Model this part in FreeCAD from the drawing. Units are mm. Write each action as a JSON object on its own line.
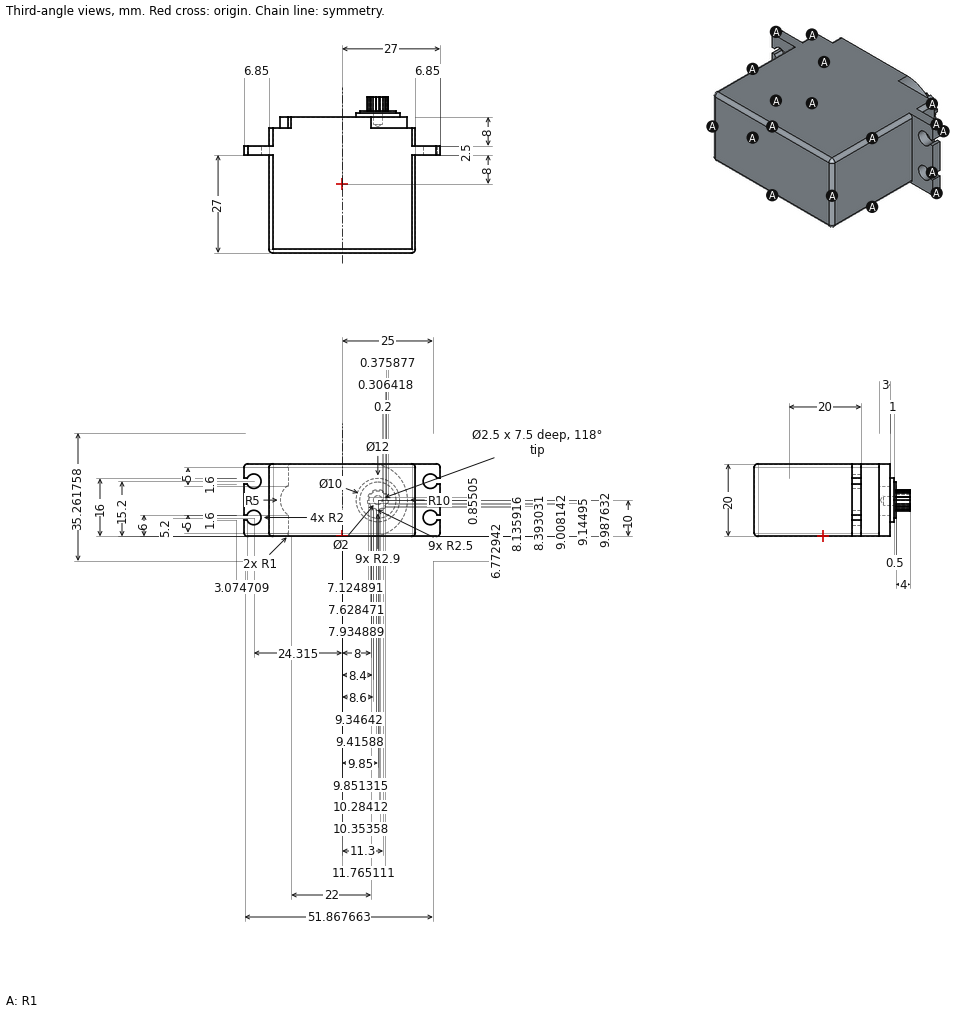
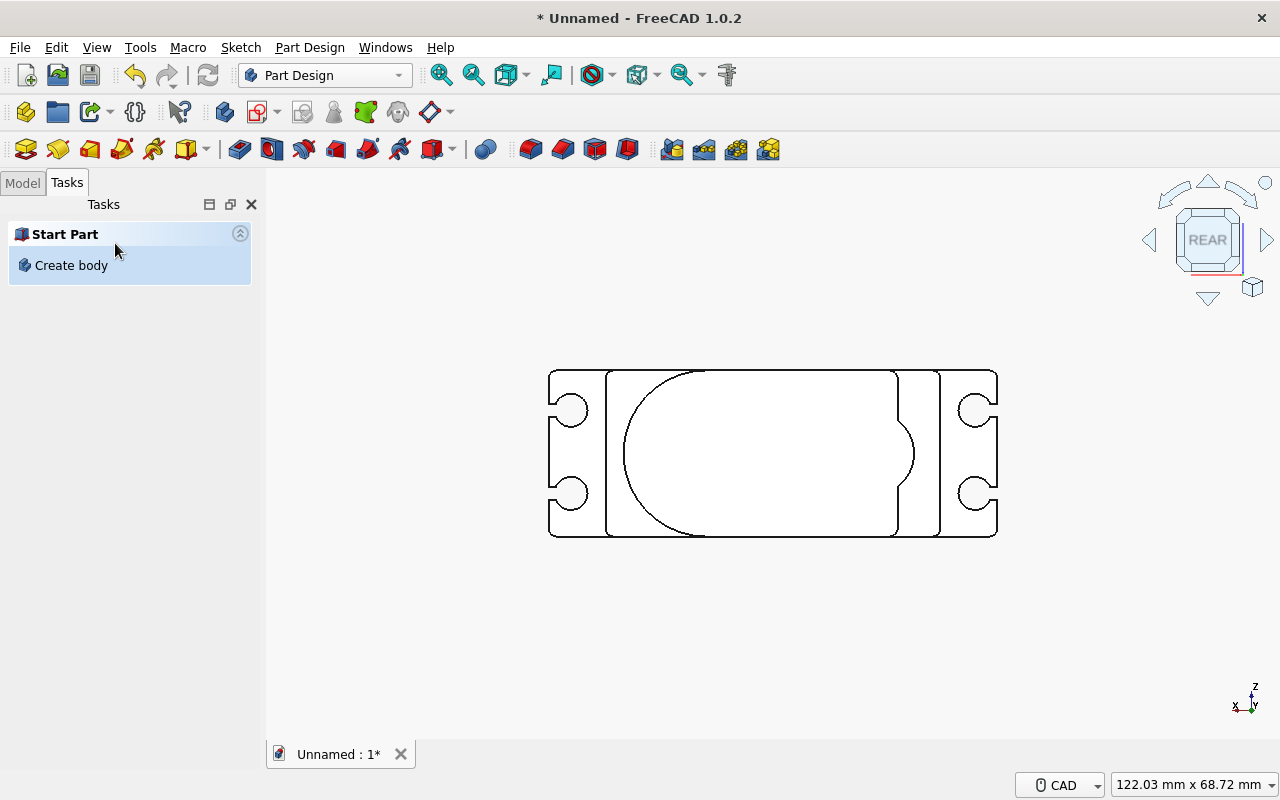
{"action": "left_click", "coordinate": [442, 76]}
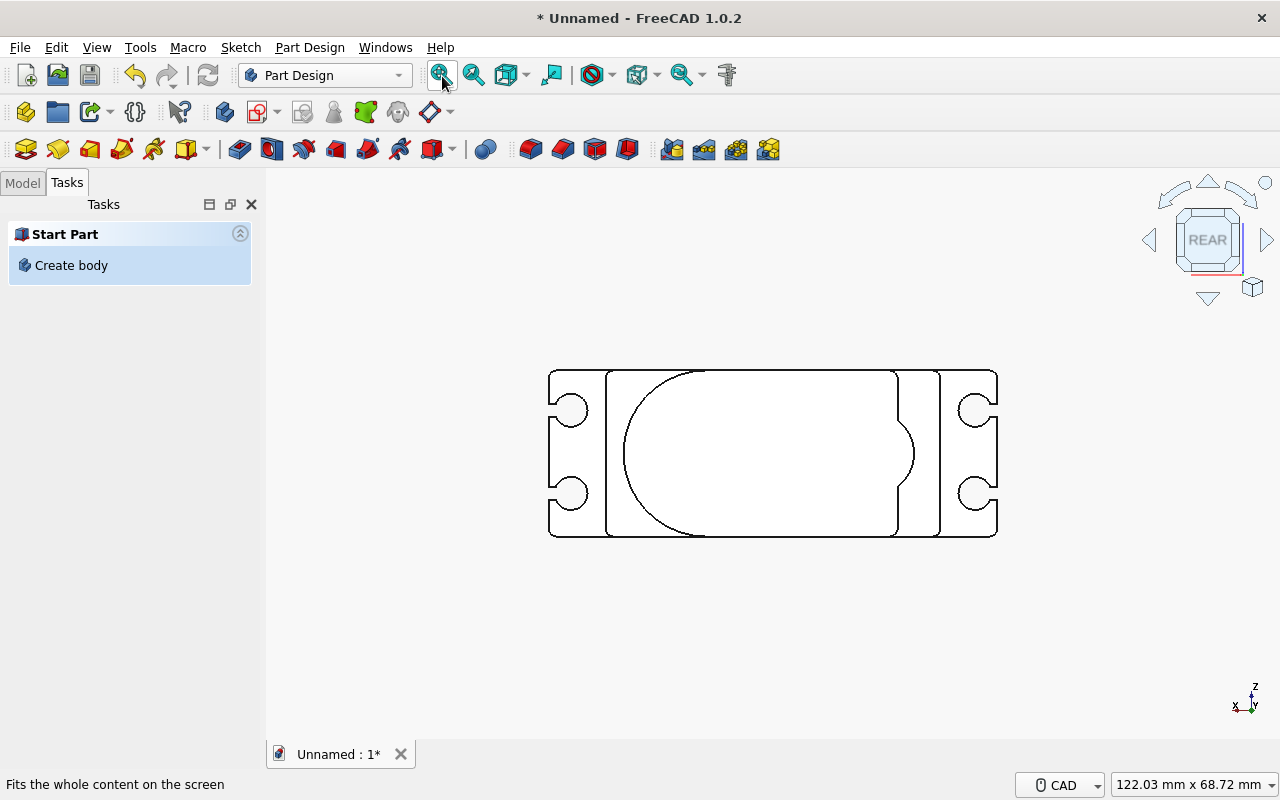
{"action": "left_click", "coordinate": [727, 452]}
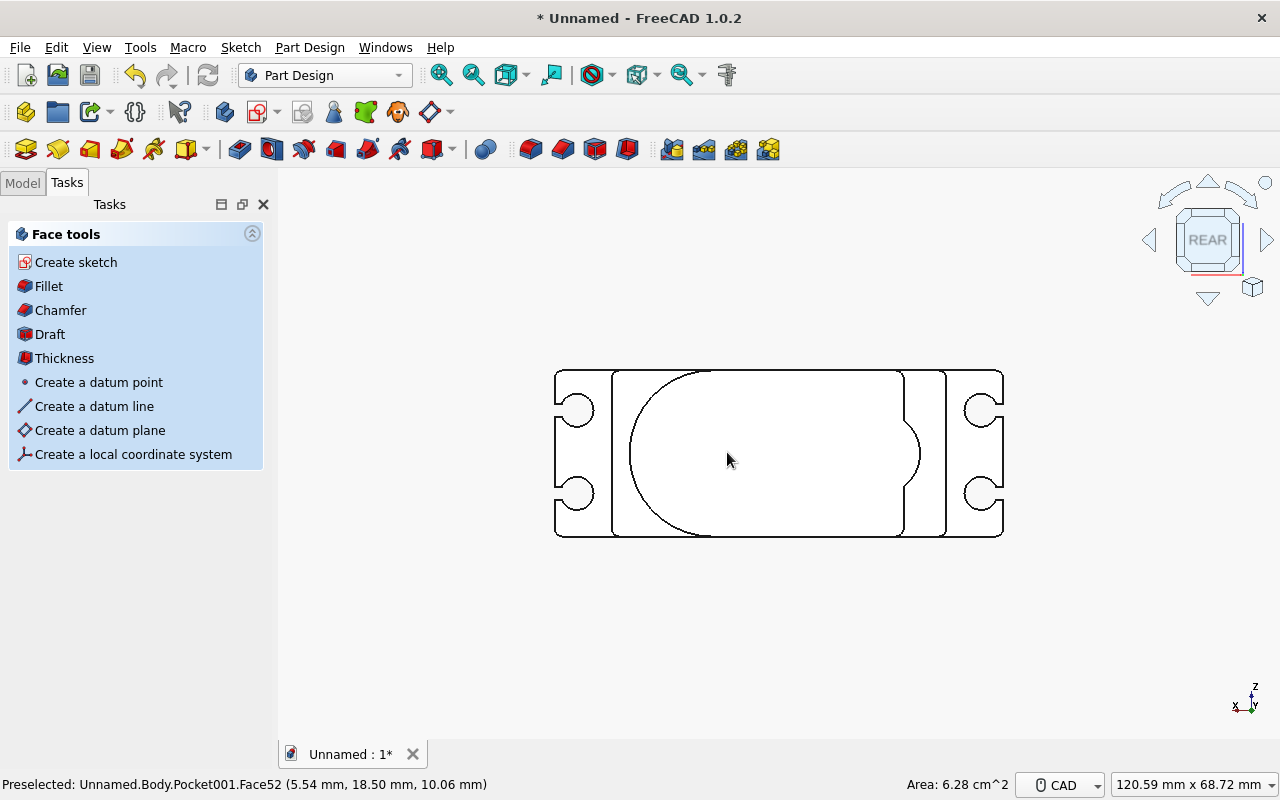
{"action": "left_click", "coordinate": [258, 112]}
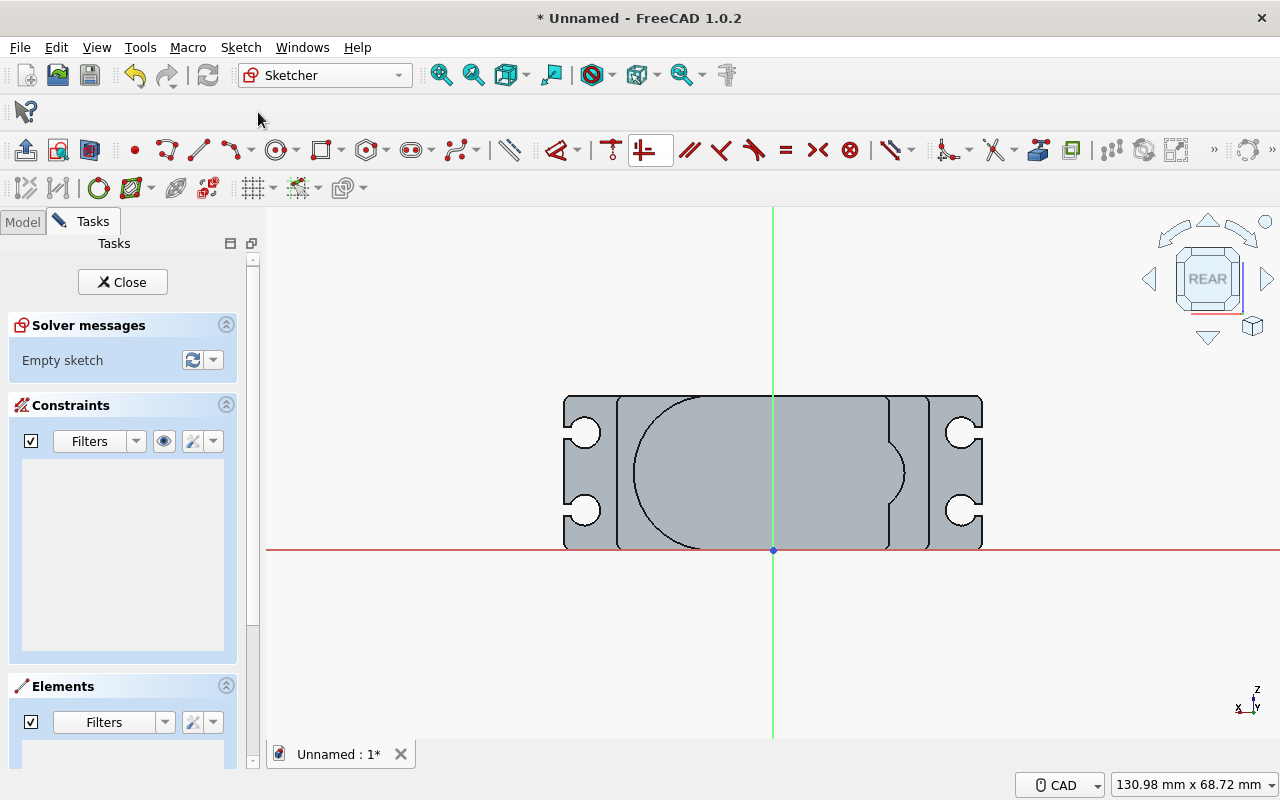
{"action": "scroll", "coordinate": [716, 497], "scroll_direction": "up", "scroll_amount": 5}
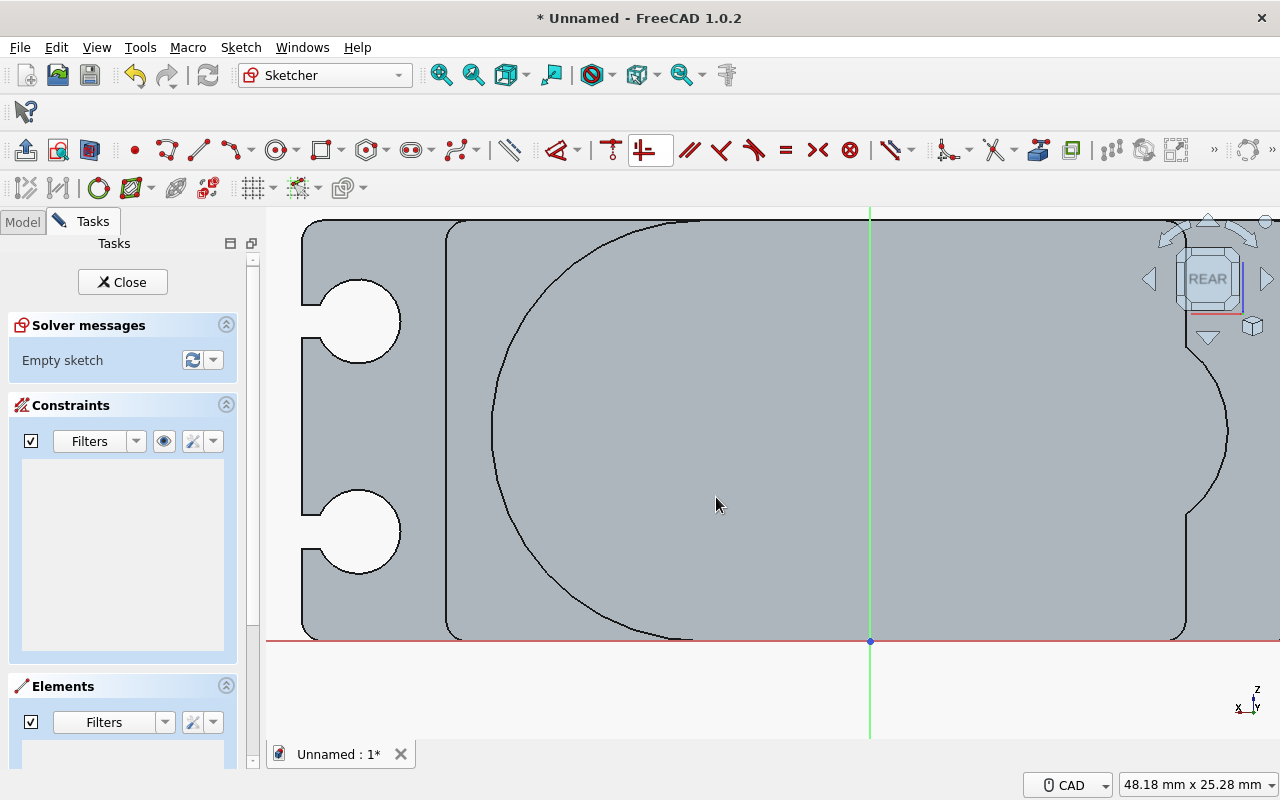
{"action": "left_click", "coordinate": [276, 150]}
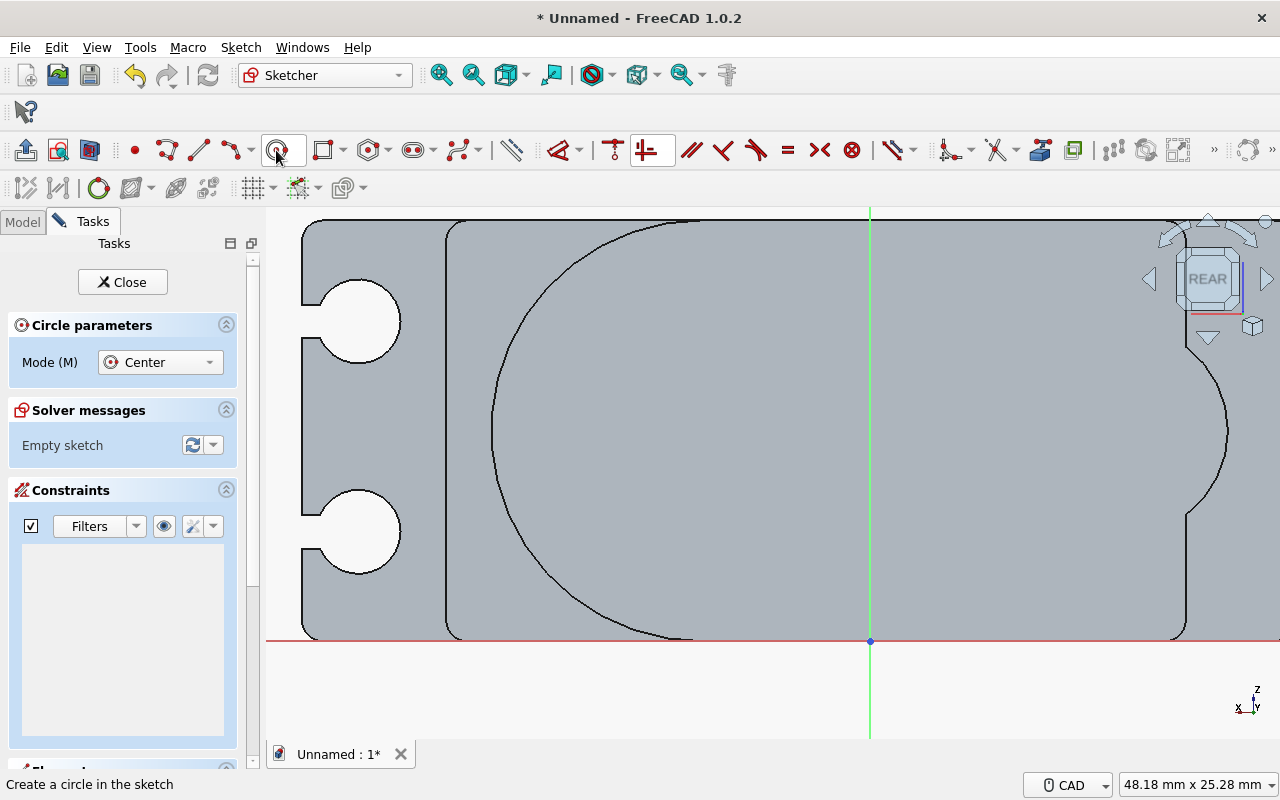
{"action": "left_click", "coordinate": [663, 431]}
{"action": "mouse_move", "coordinate": [752, 342]}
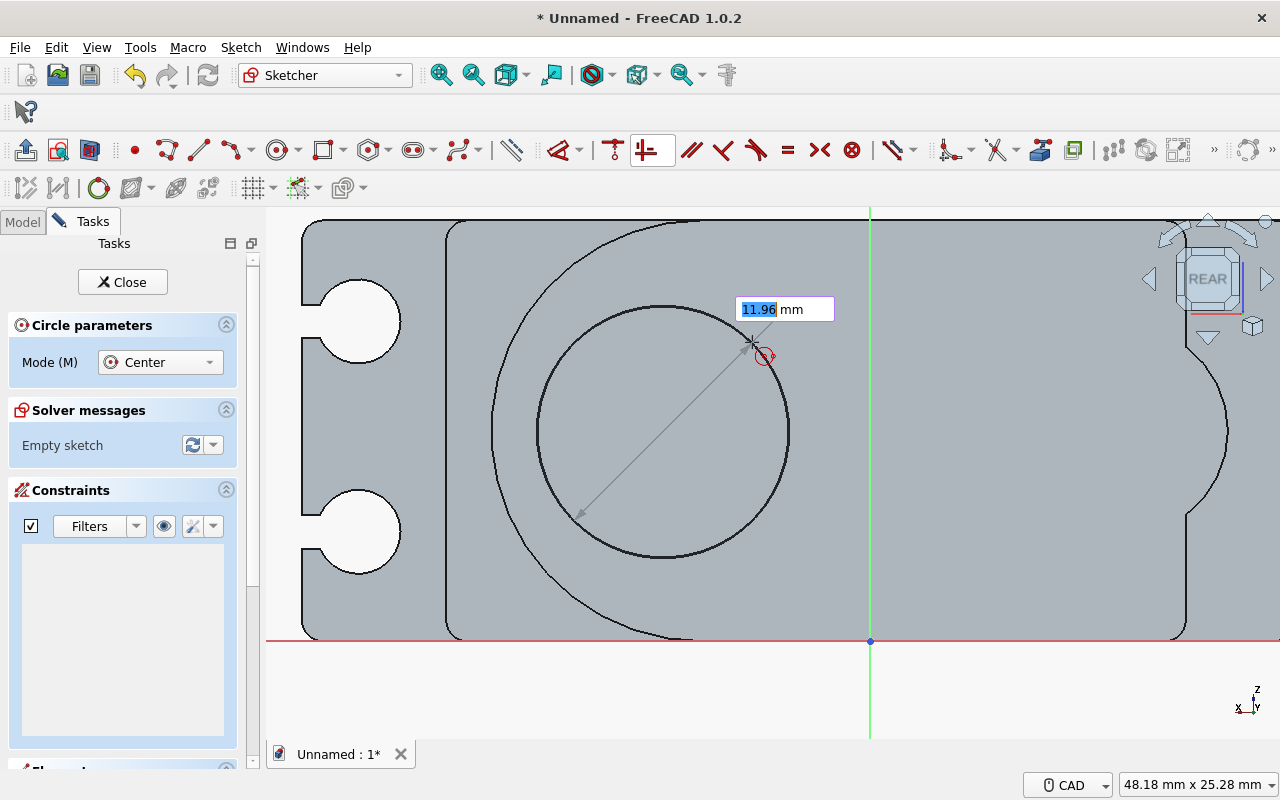
{"action": "type", "text": "12"}
{"action": "key", "text": "Return"}
{"action": "key", "text": "Escape"}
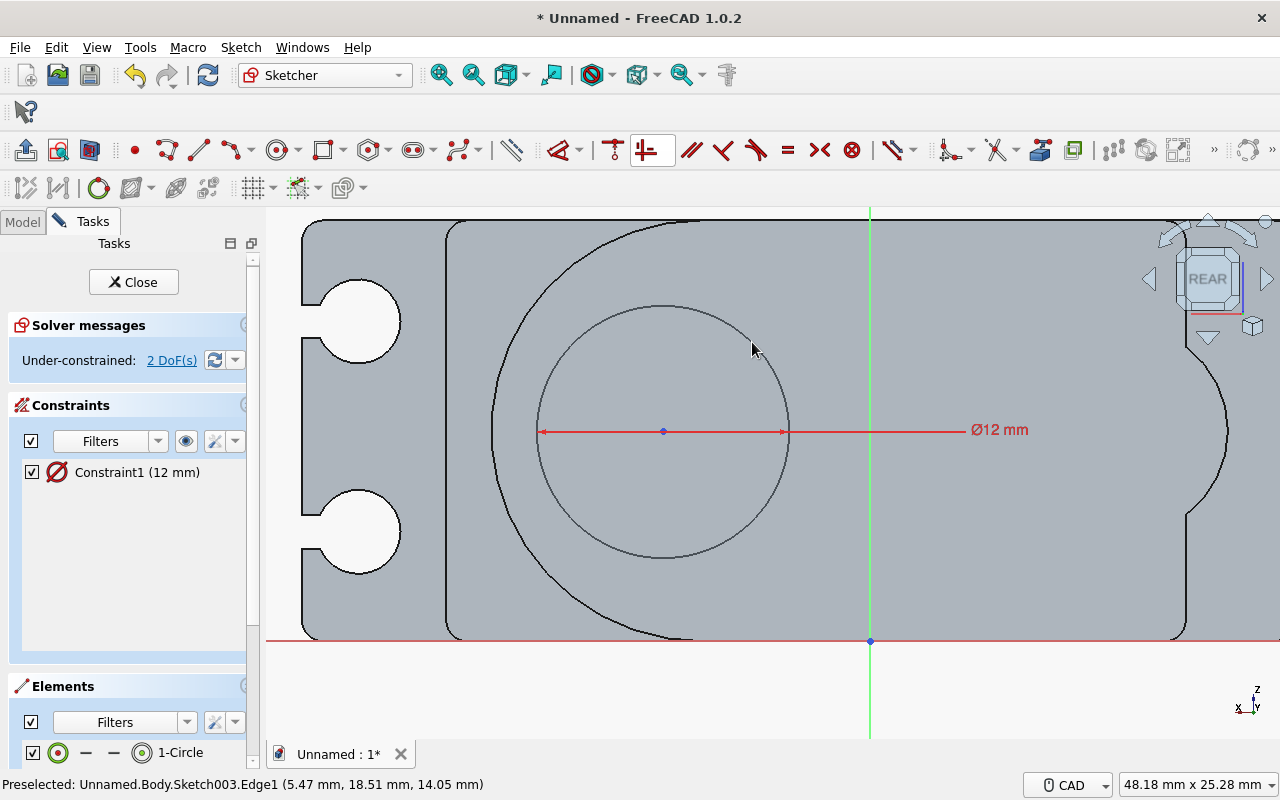
{"action": "left_click", "coordinate": [558, 150]}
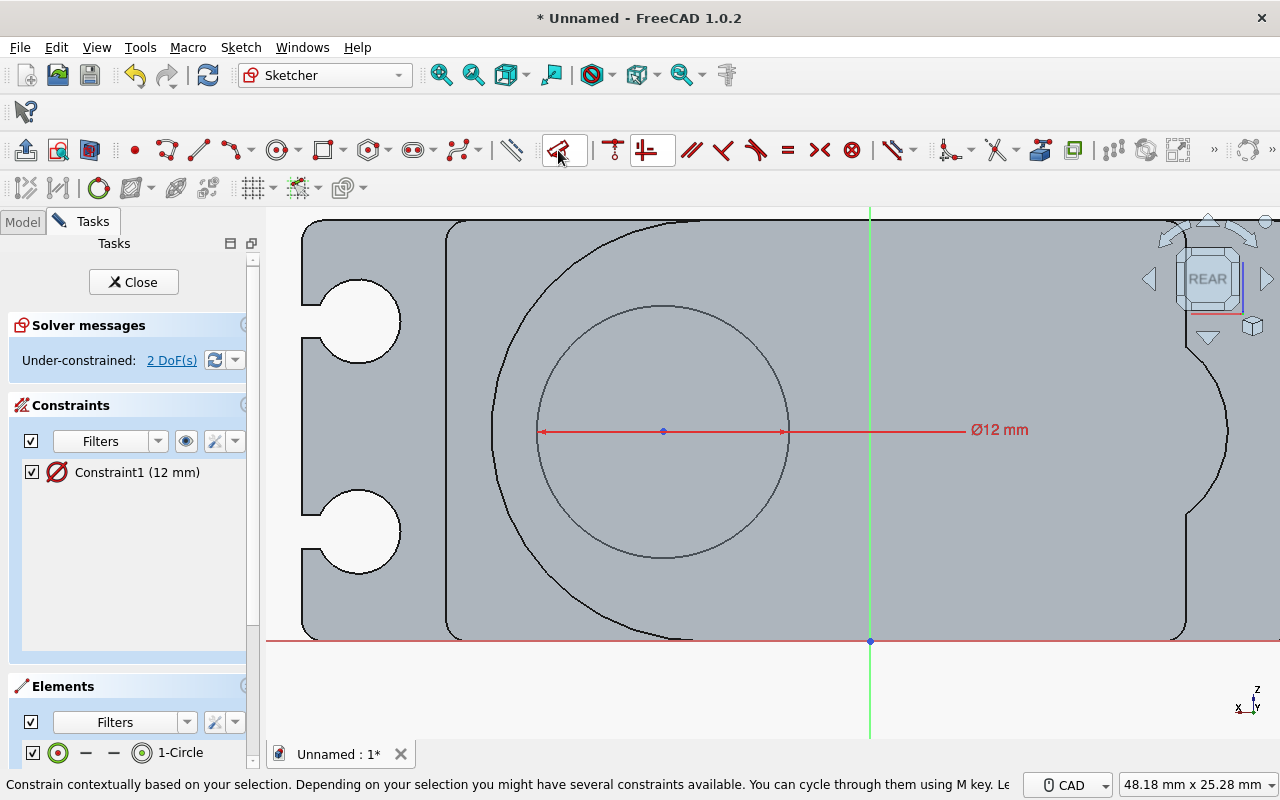
{"action": "left_click", "coordinate": [663, 432]}
{"action": "left_click", "coordinate": [904, 537]}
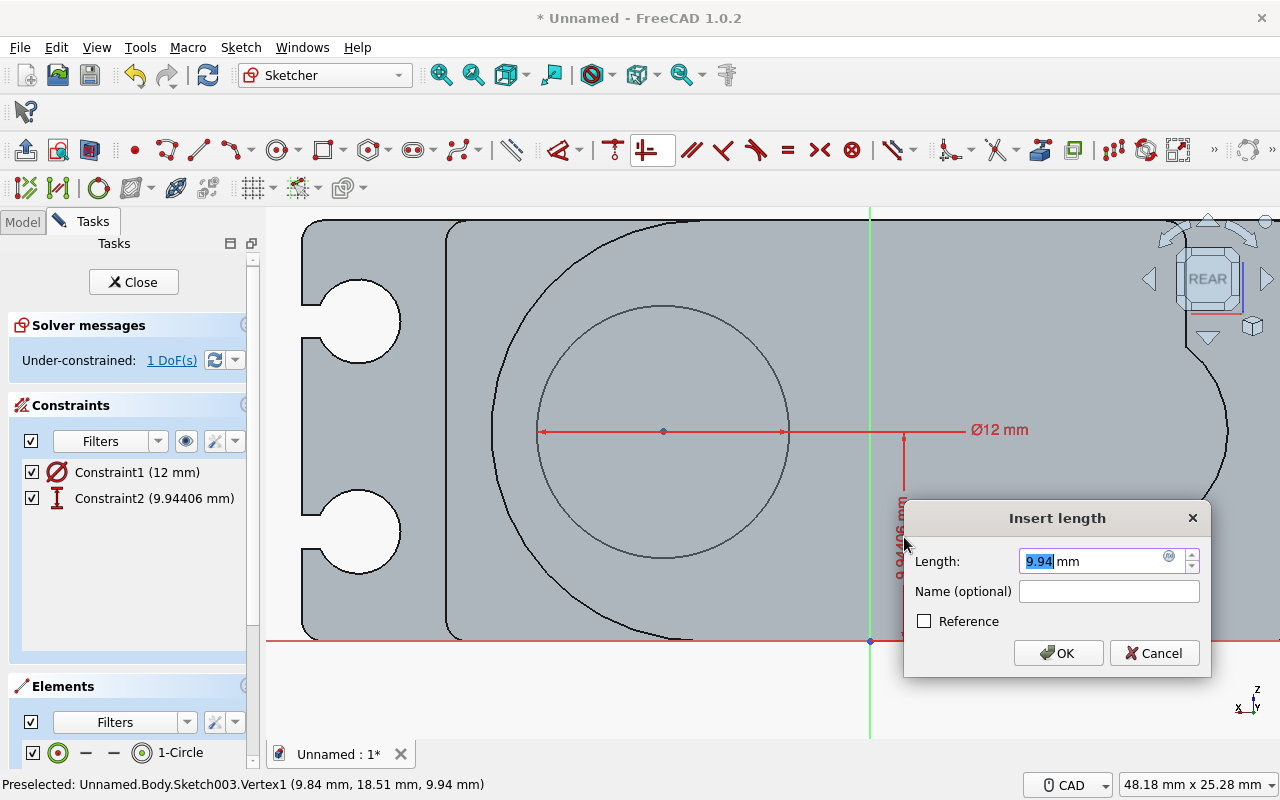
{"action": "type", "text": "10"}
{"action": "key", "text": "Return"}